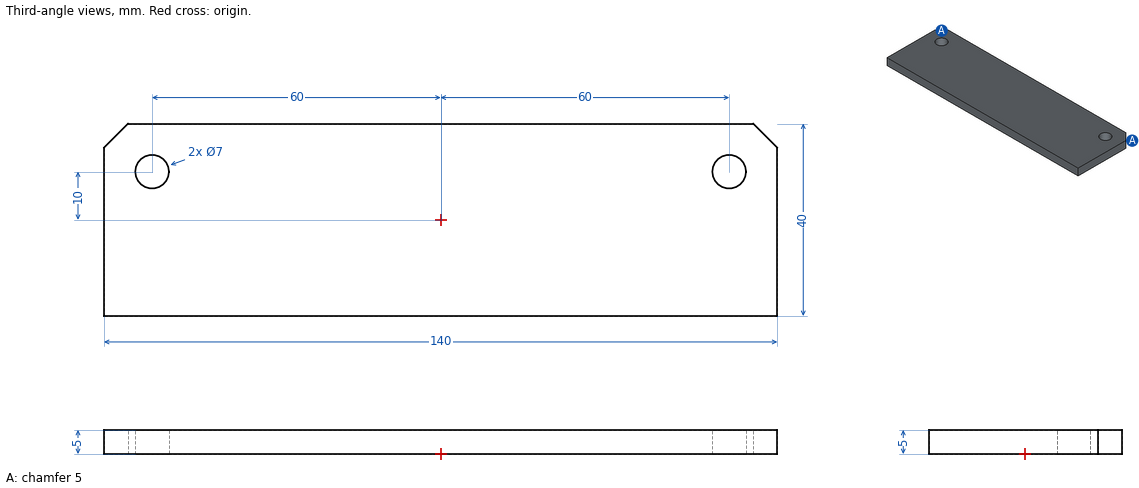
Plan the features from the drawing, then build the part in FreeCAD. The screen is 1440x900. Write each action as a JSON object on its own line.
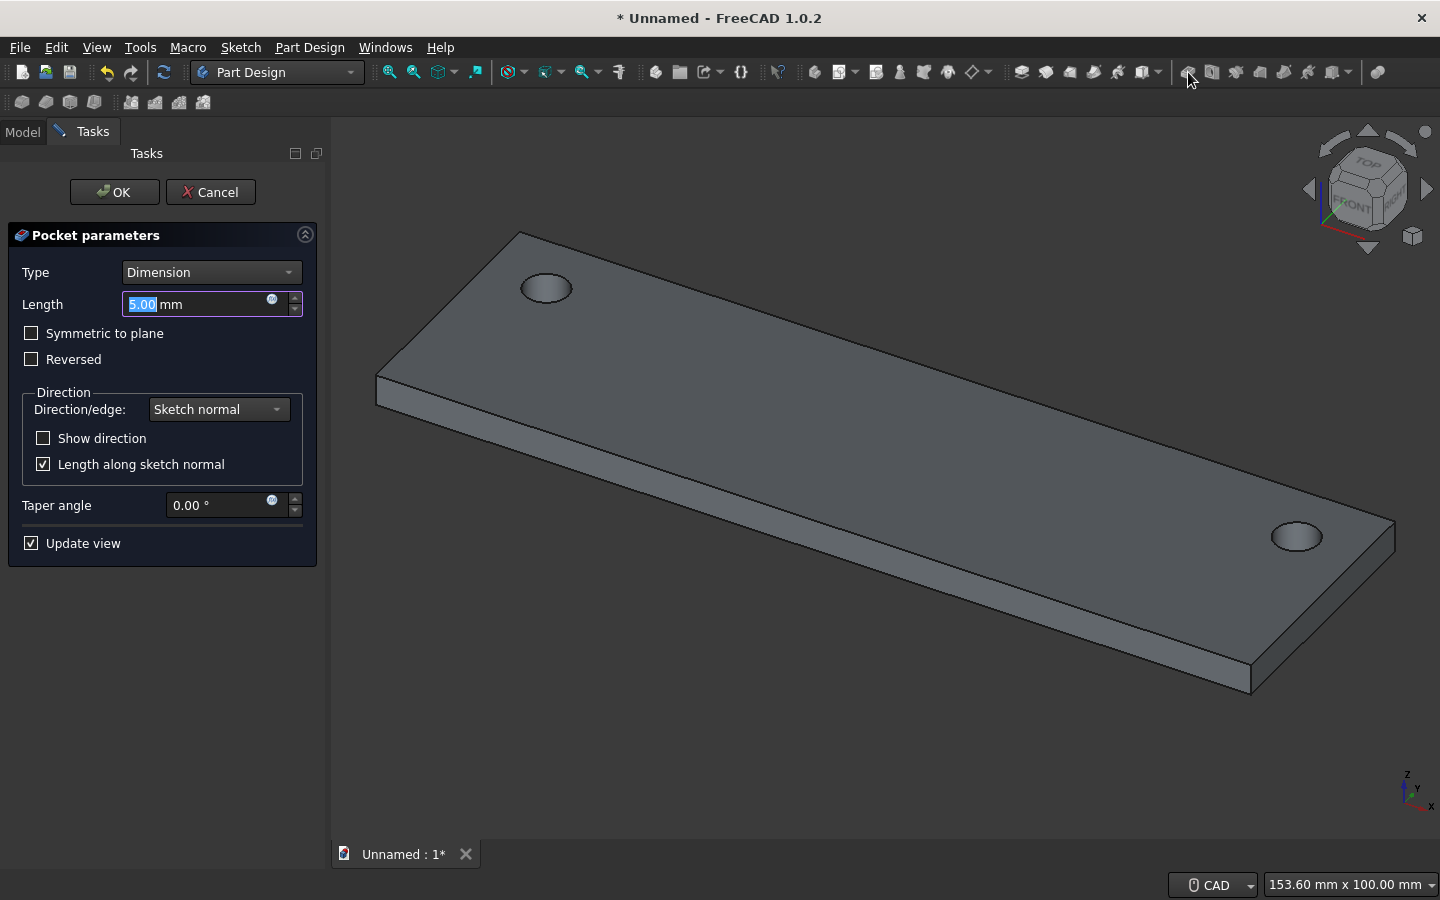
{"action": "type", "text": "5"}
{"action": "key", "text": "Tab"}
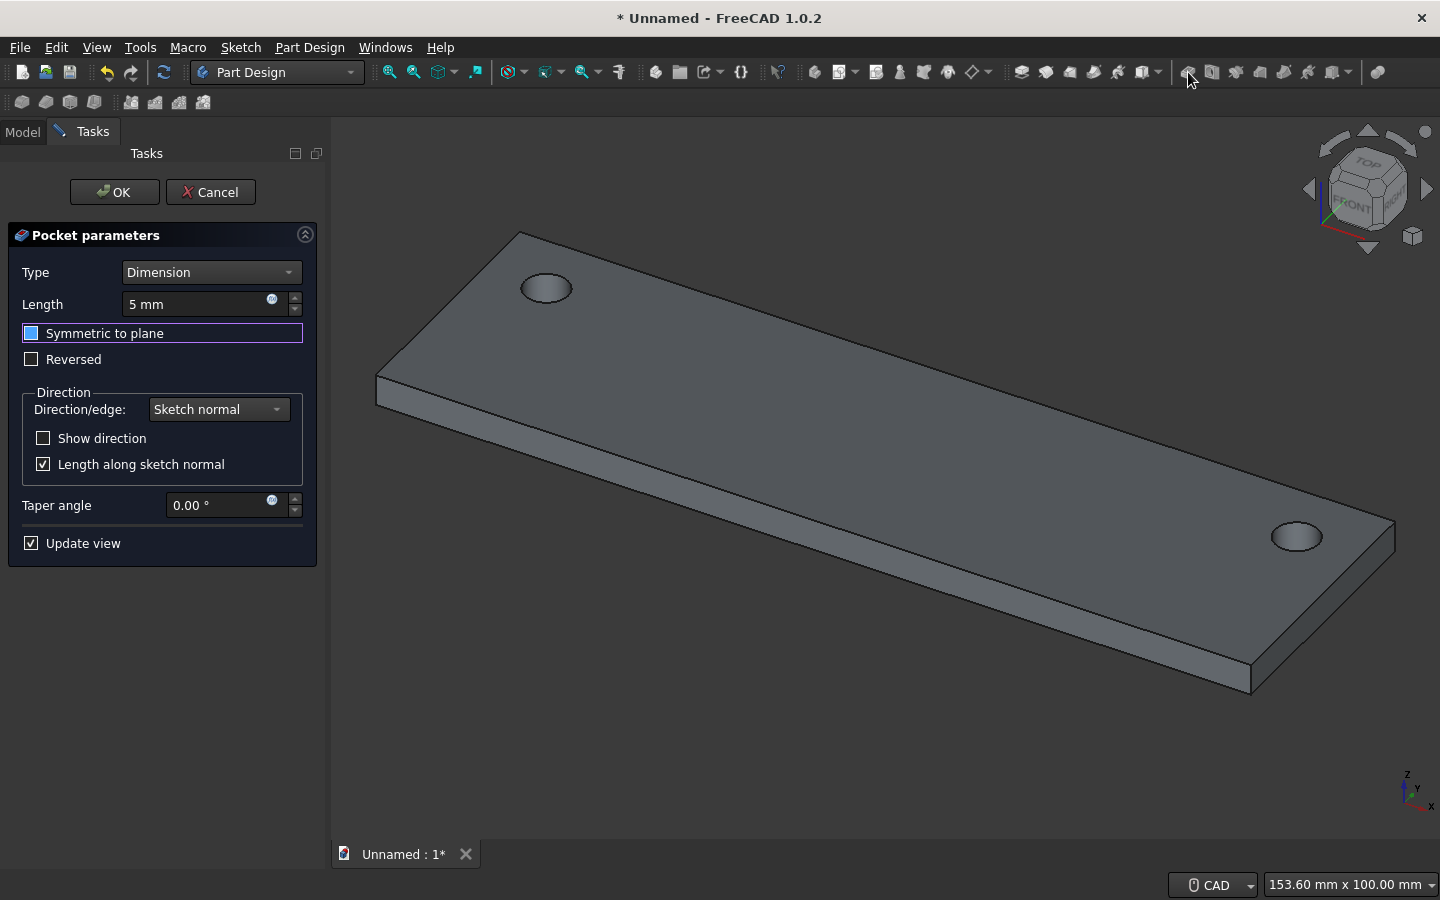
{"action": "left_click", "coordinate": [115, 192]}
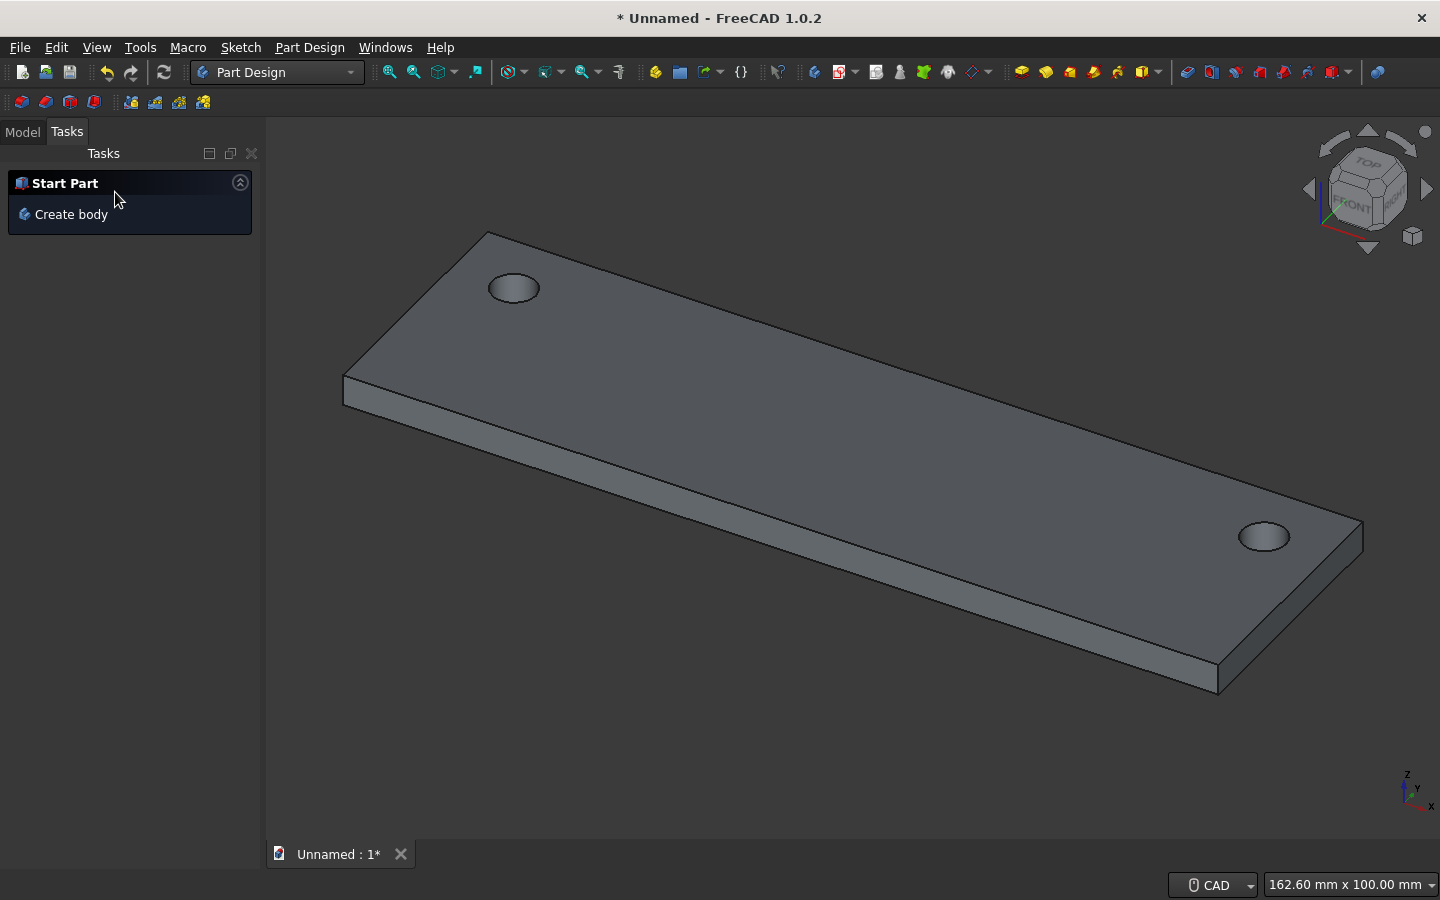
{"action": "key", "text": "0"}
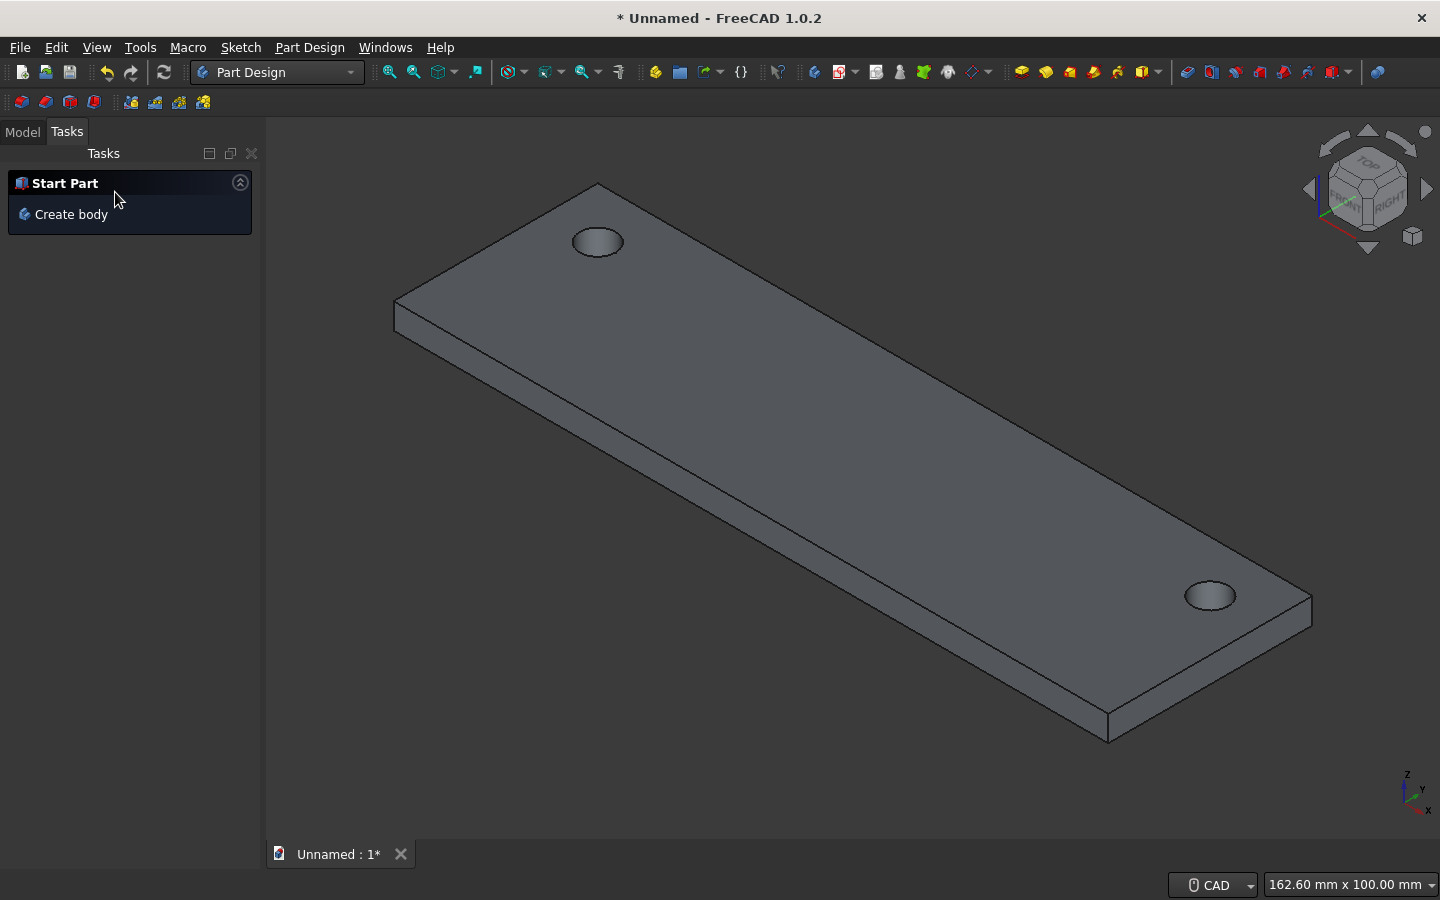
{"action": "key", "text": "2"}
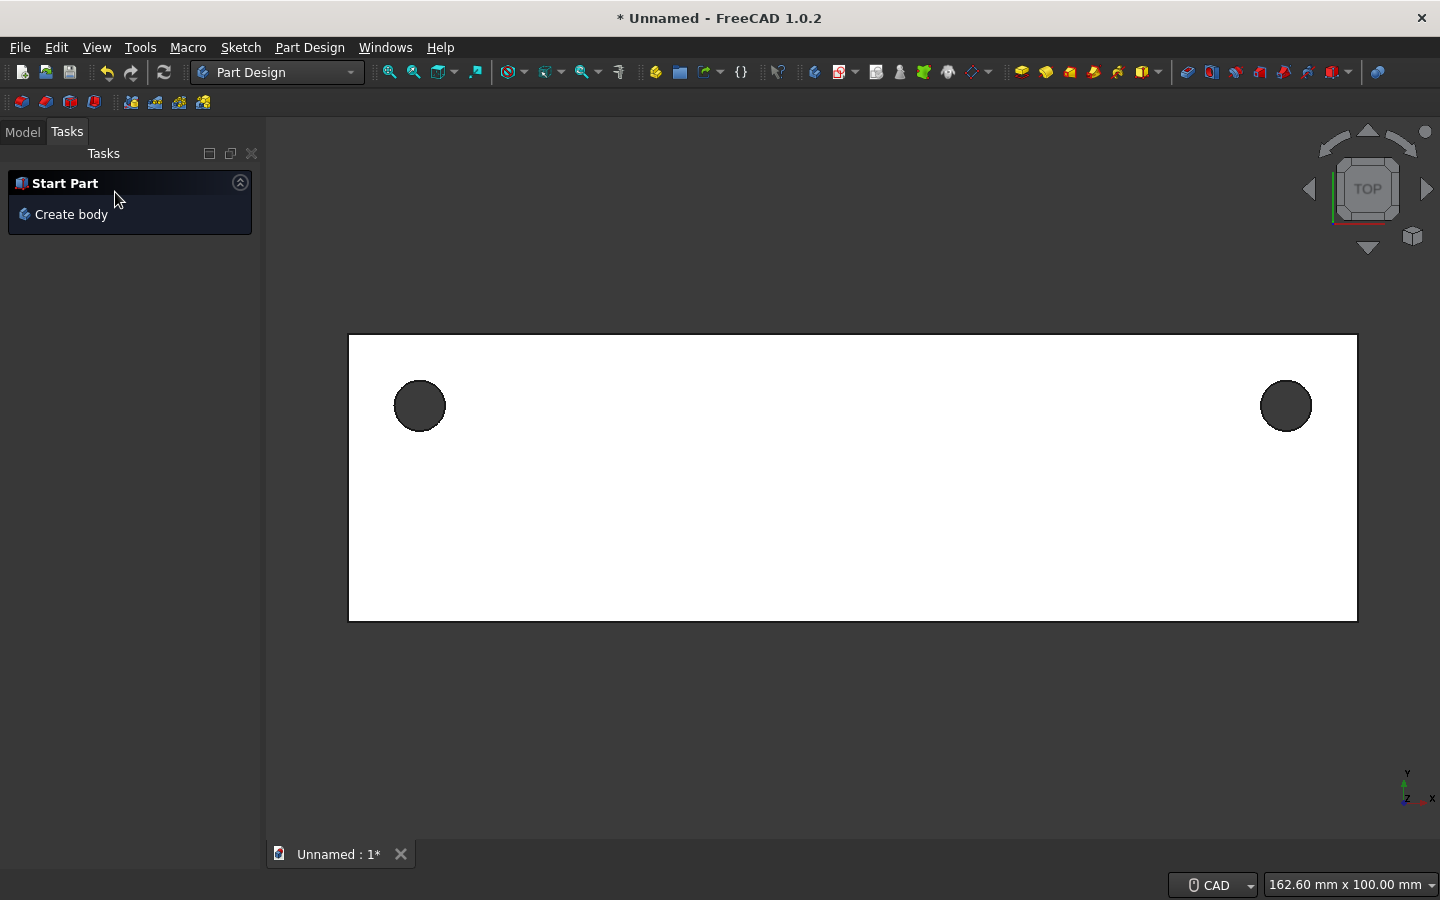
{"action": "key", "text": "1"}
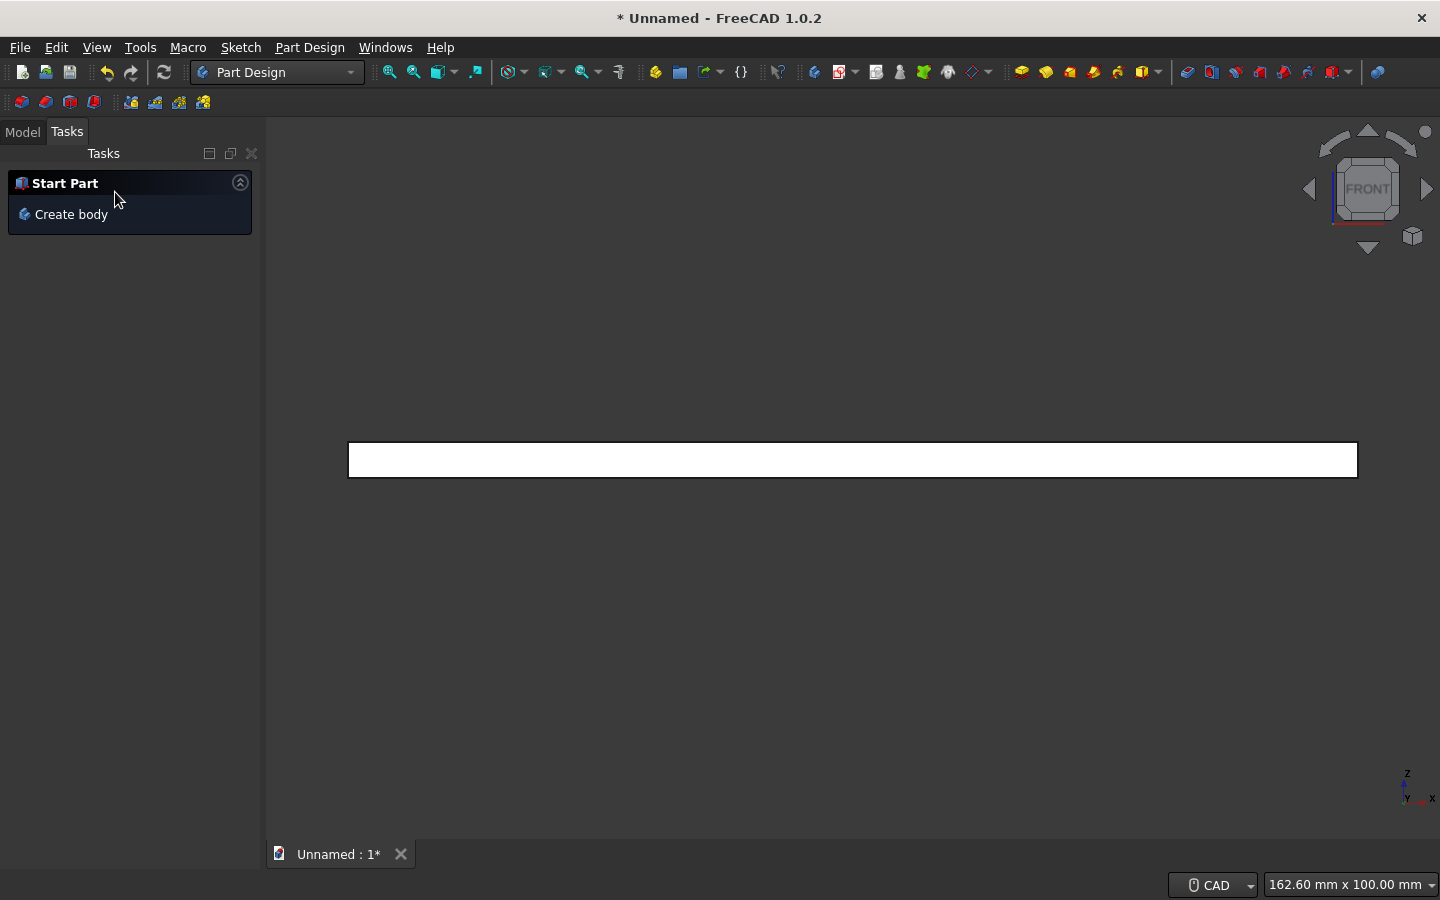
{"action": "key", "text": "3"}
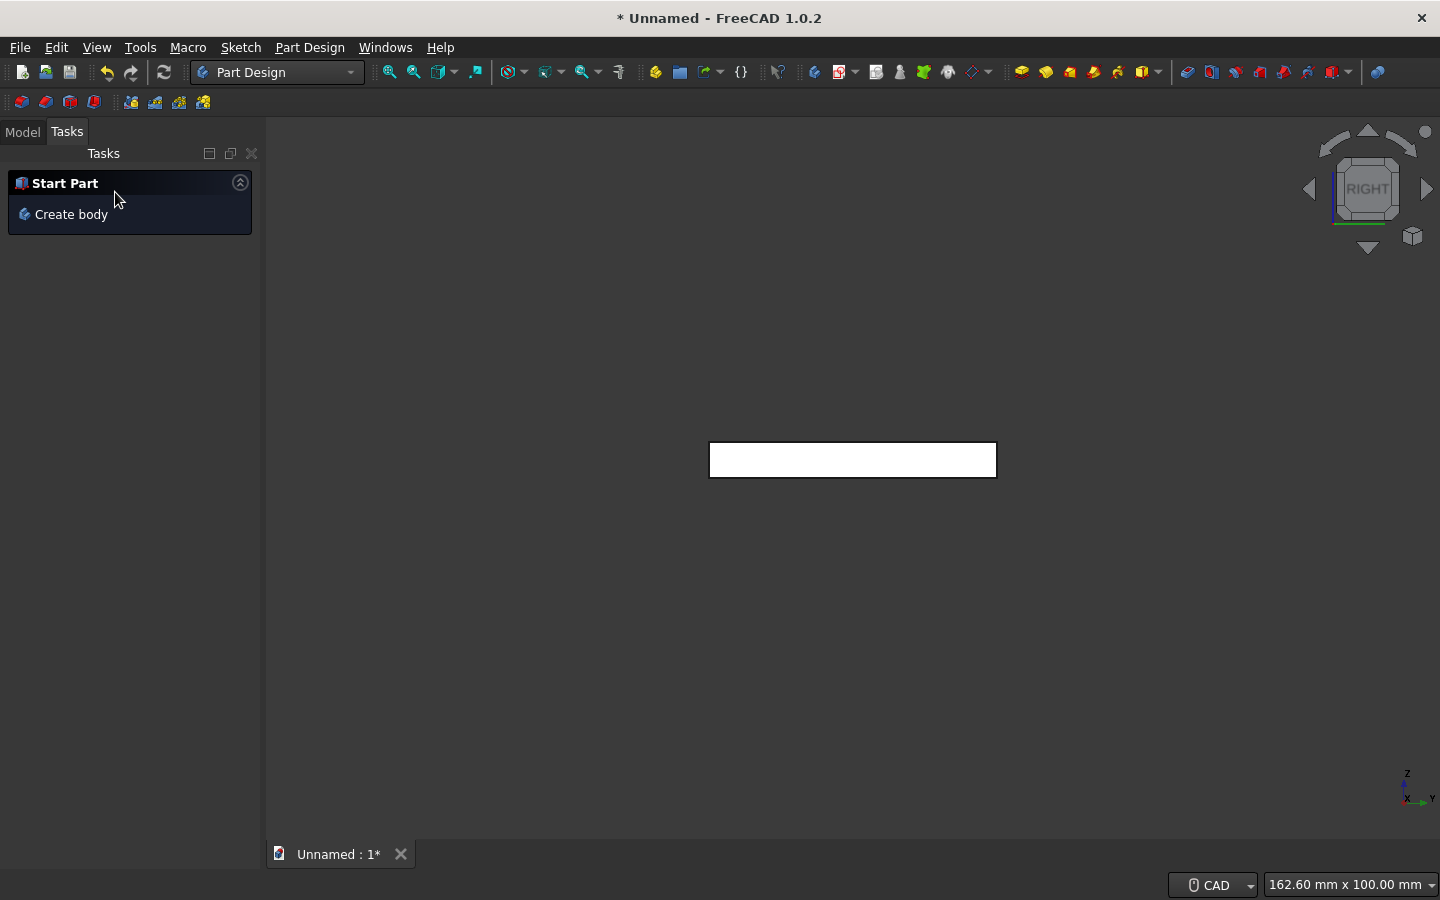
{"action": "left_click", "coordinate": [390, 72]}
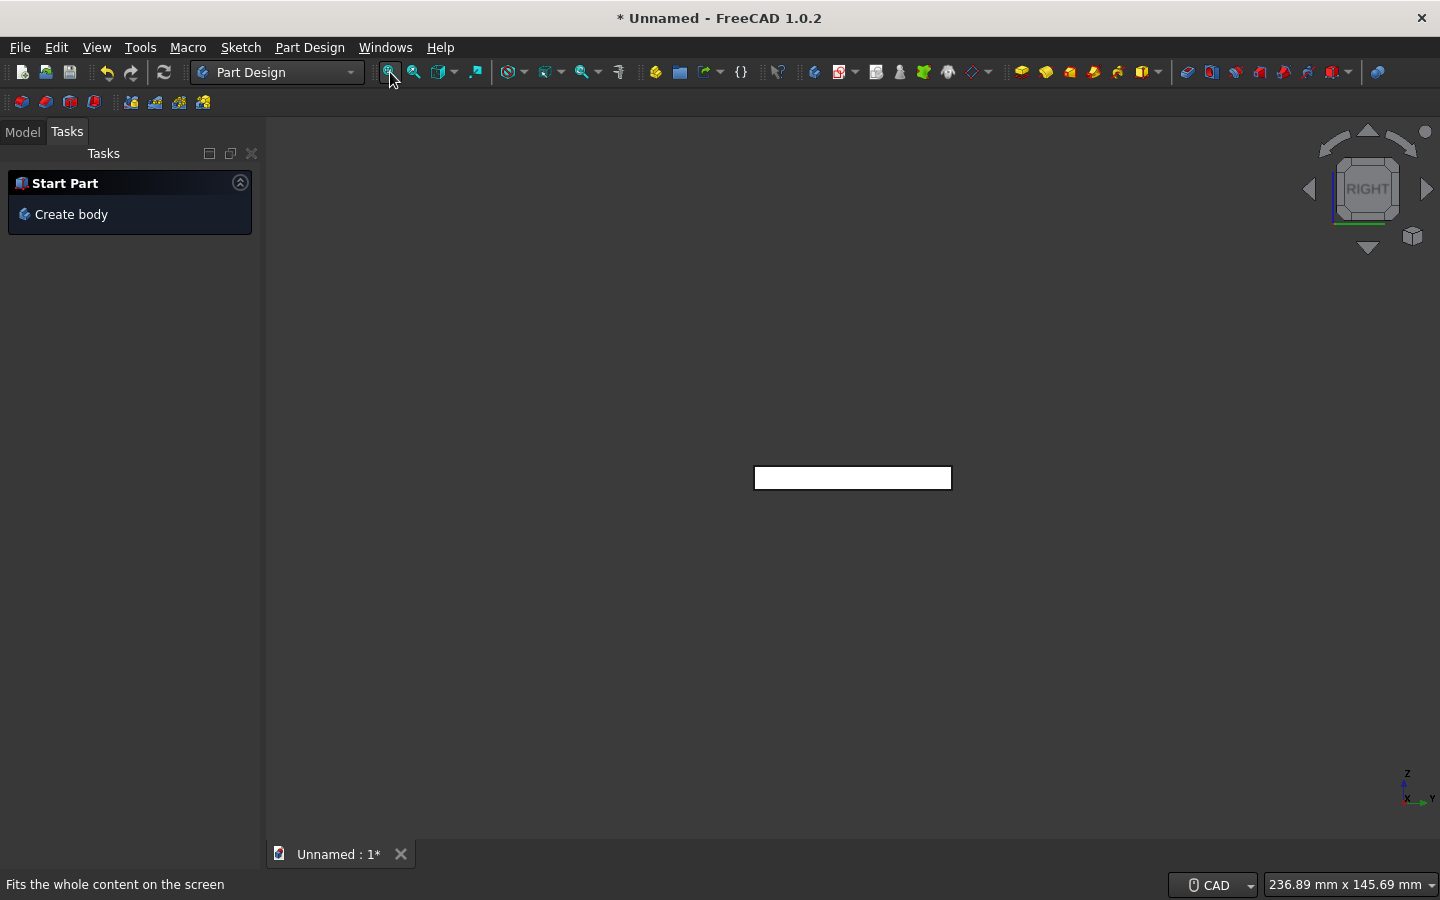
{"action": "left_click", "coordinate": [952, 477]}